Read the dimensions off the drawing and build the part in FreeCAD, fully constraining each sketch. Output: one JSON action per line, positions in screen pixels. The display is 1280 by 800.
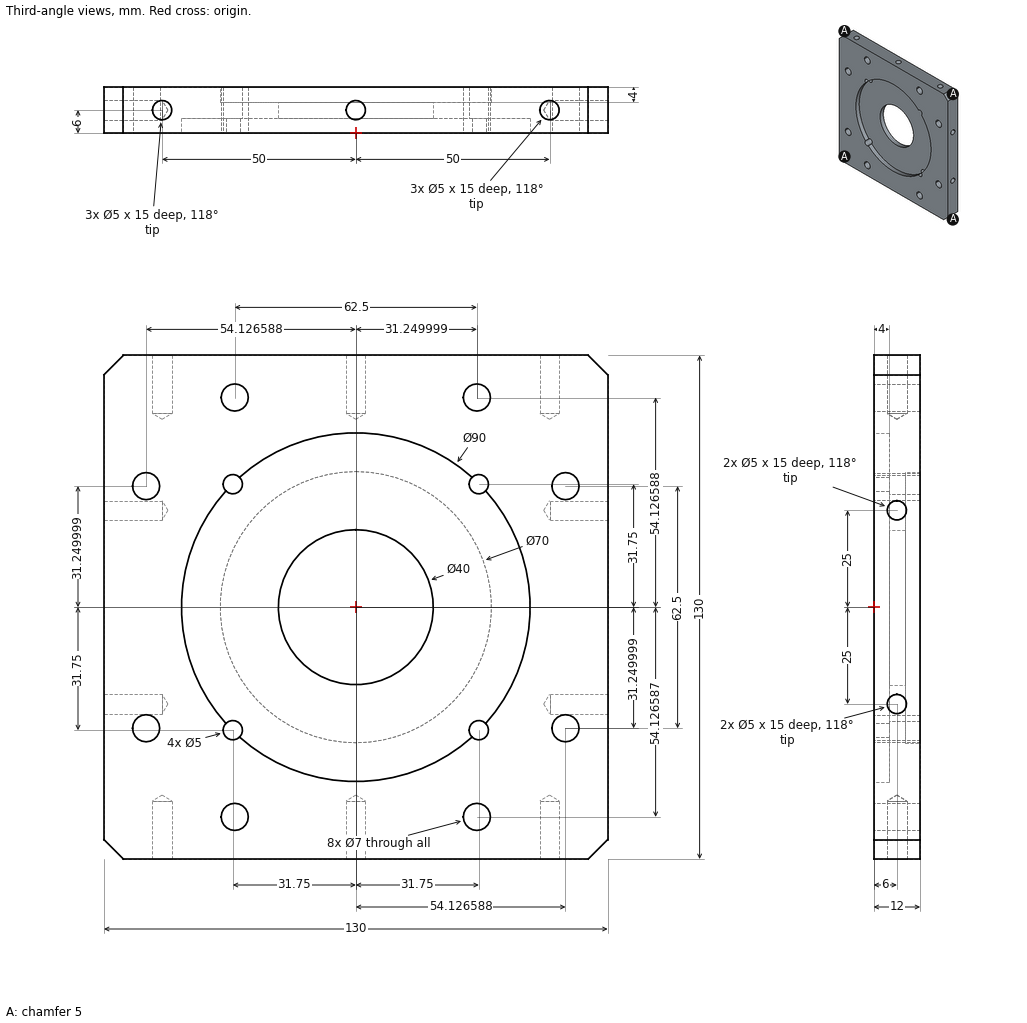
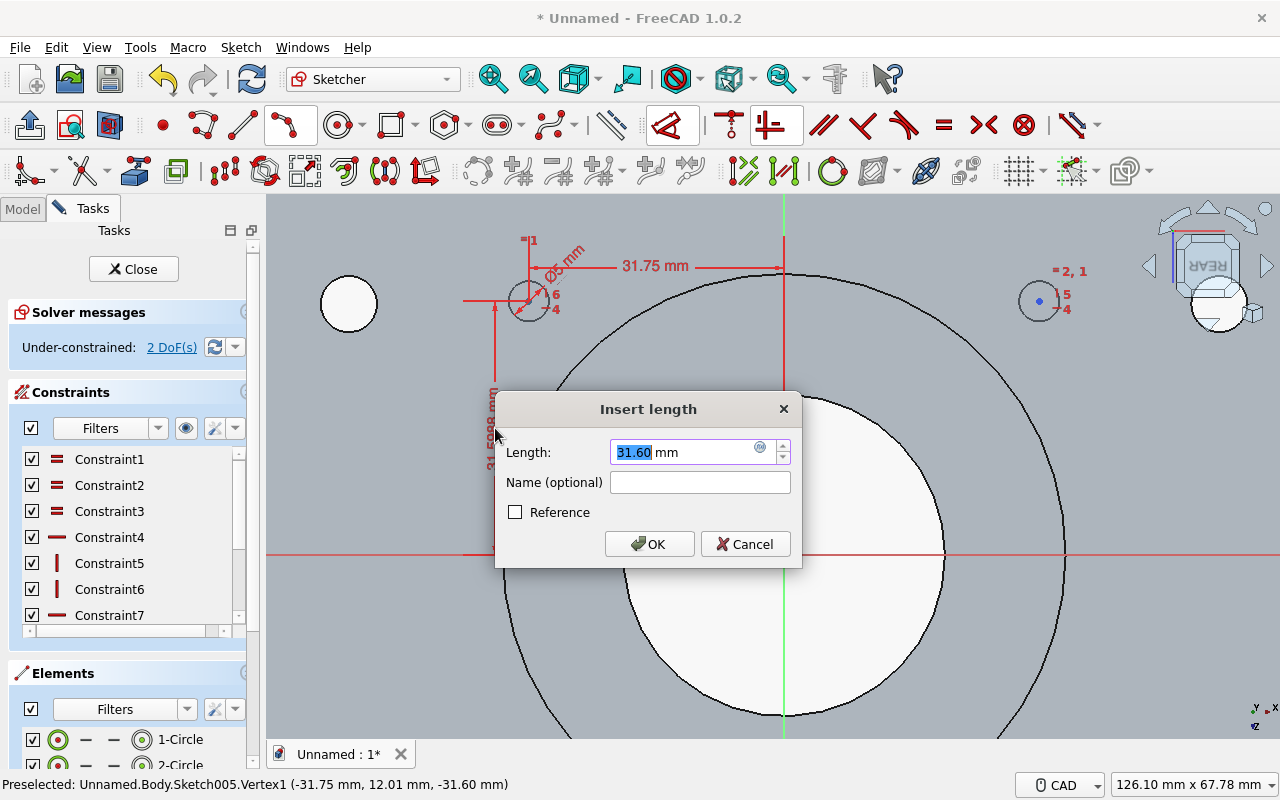
{"action": "type", "text": "31.75"}
{"action": "key", "text": "Return"}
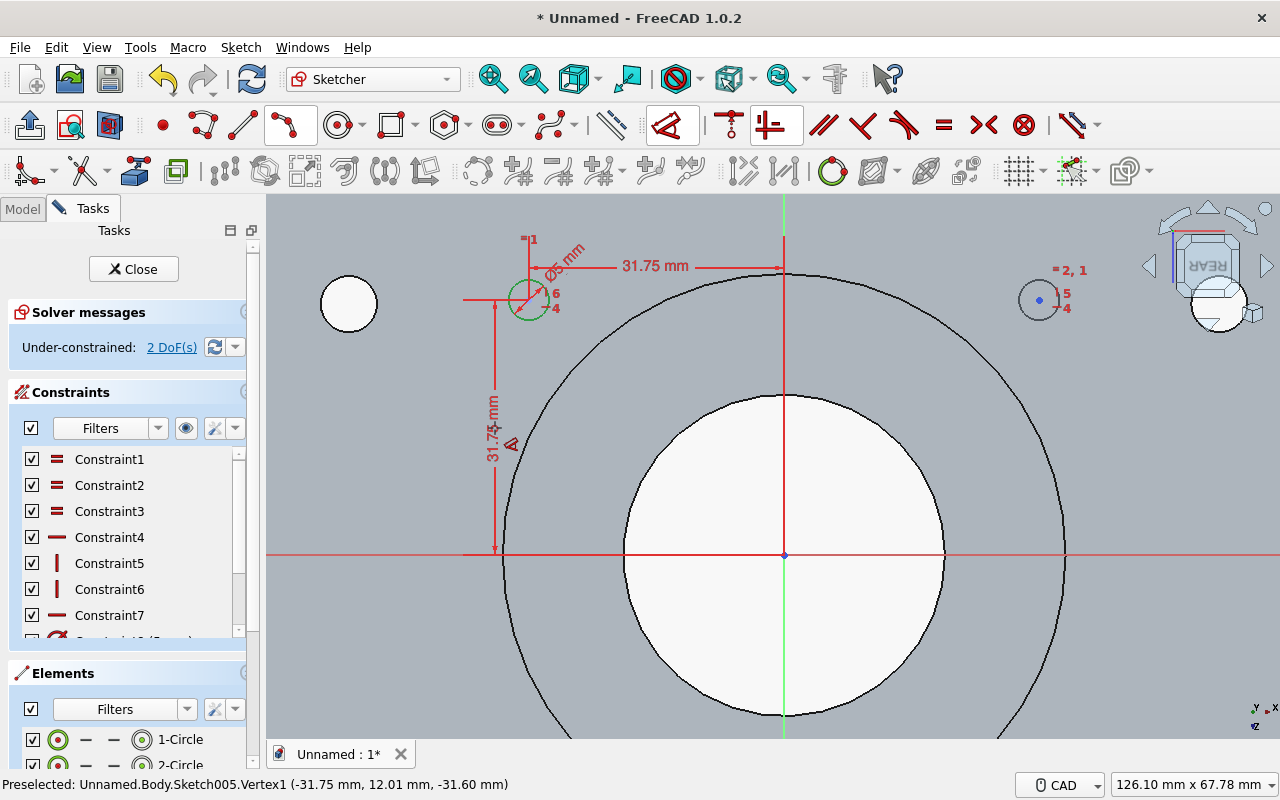
{"action": "left_click", "coordinate": [1039, 300]}
{"action": "left_click", "coordinate": [912, 266]}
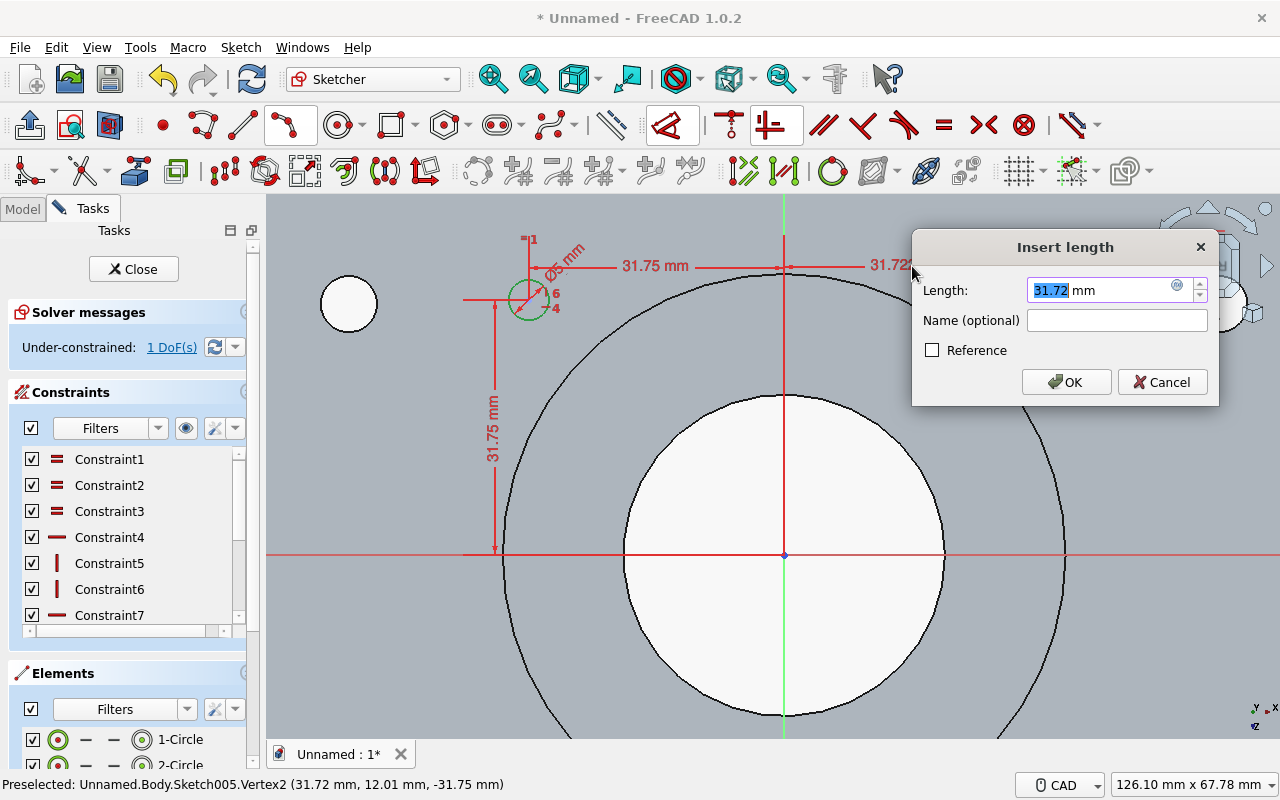
{"action": "type", "text": "31.75"}
{"action": "key", "text": "Return"}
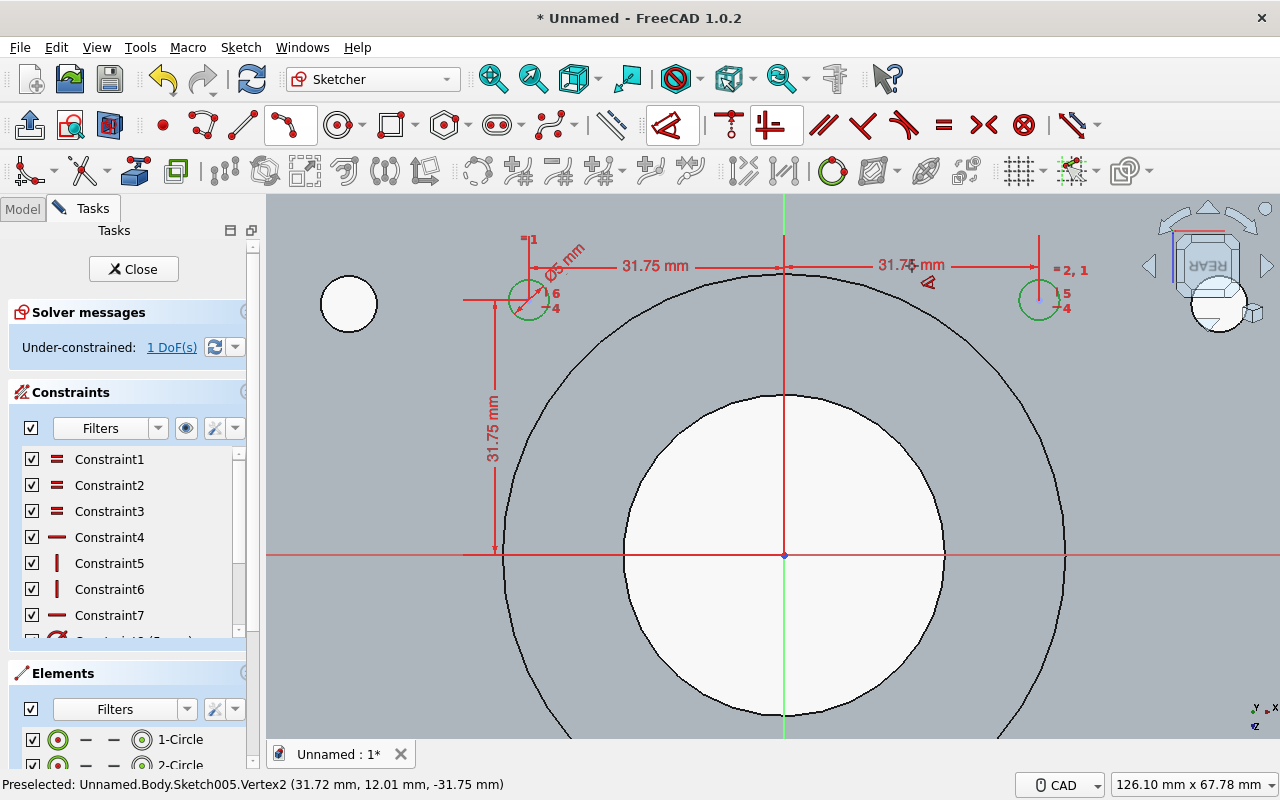
{"action": "scroll", "coordinate": [543, 286], "scroll_direction": "down", "scroll_amount": 2}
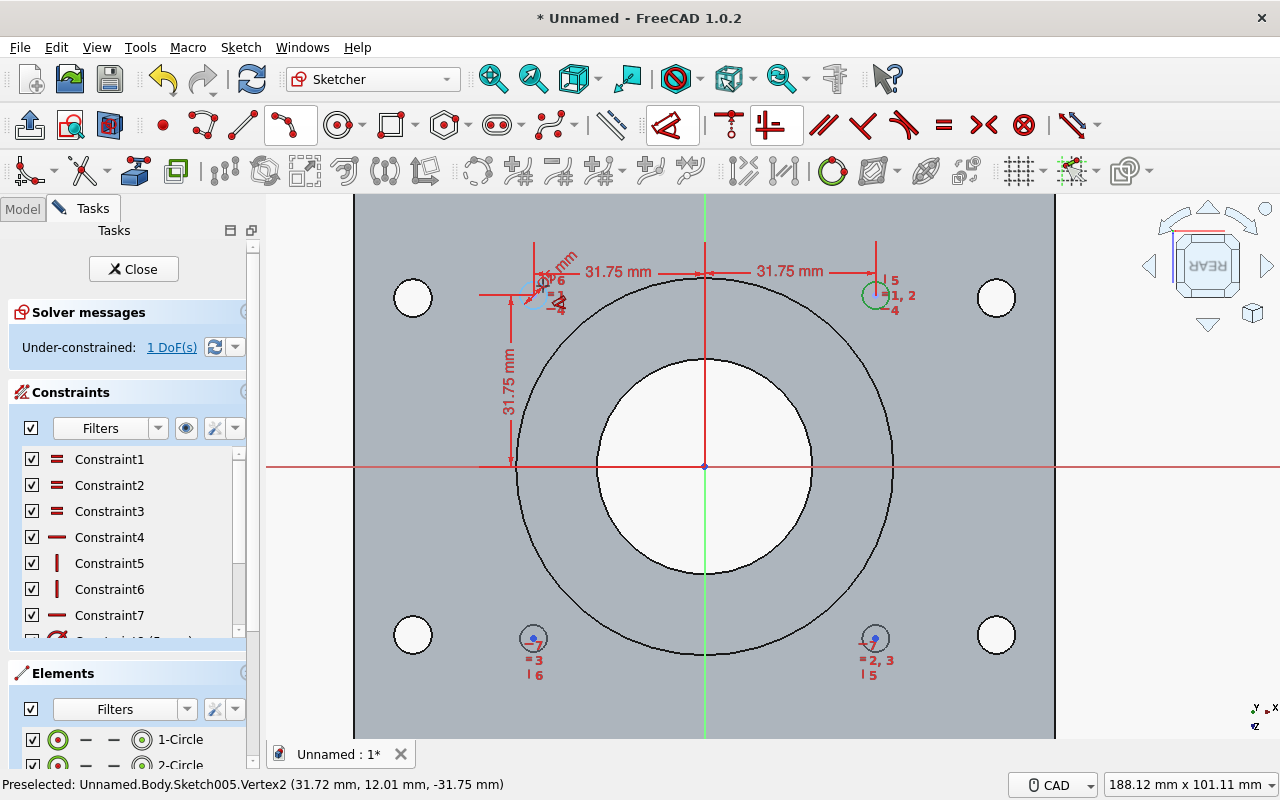
{"action": "left_click", "coordinate": [876, 638]}
{"action": "left_click", "coordinate": [910, 553]}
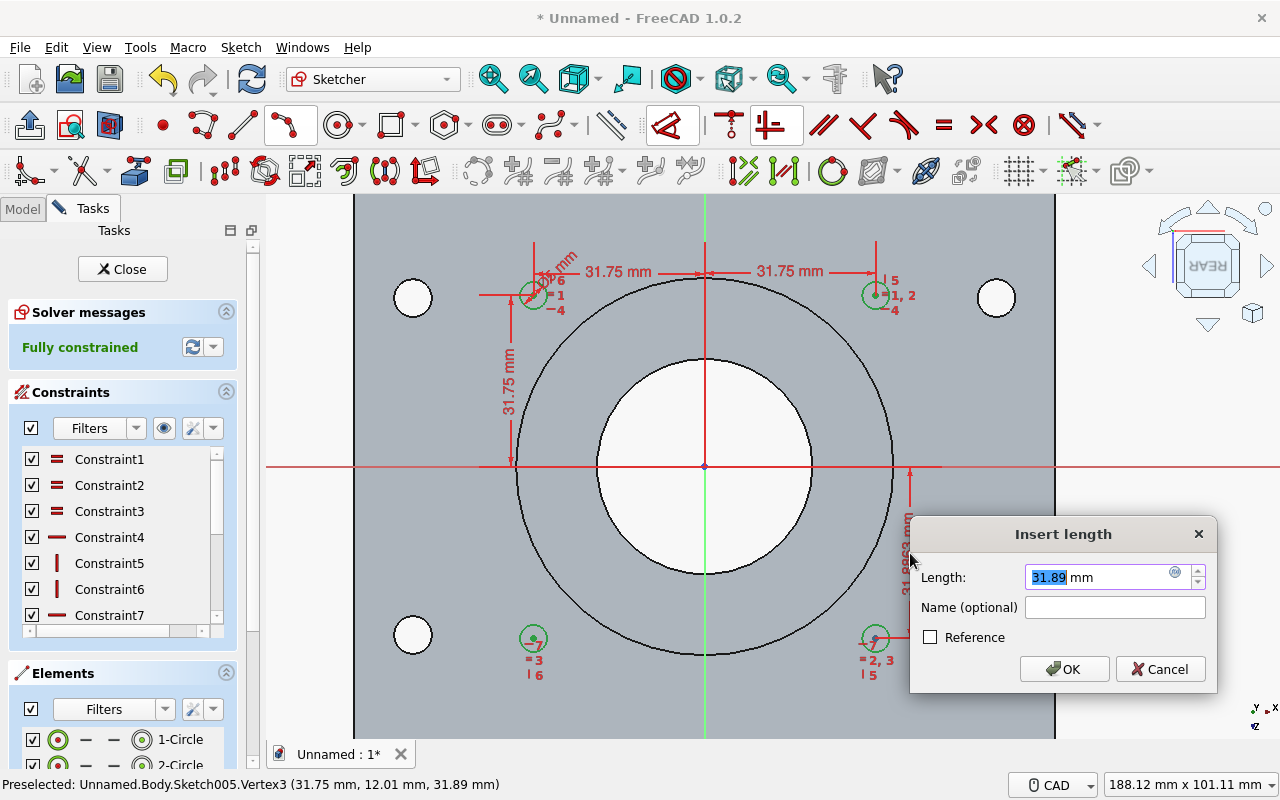
{"action": "type", "text": "31.75"}
{"action": "key", "text": "Return"}
{"action": "key", "text": "Escape"}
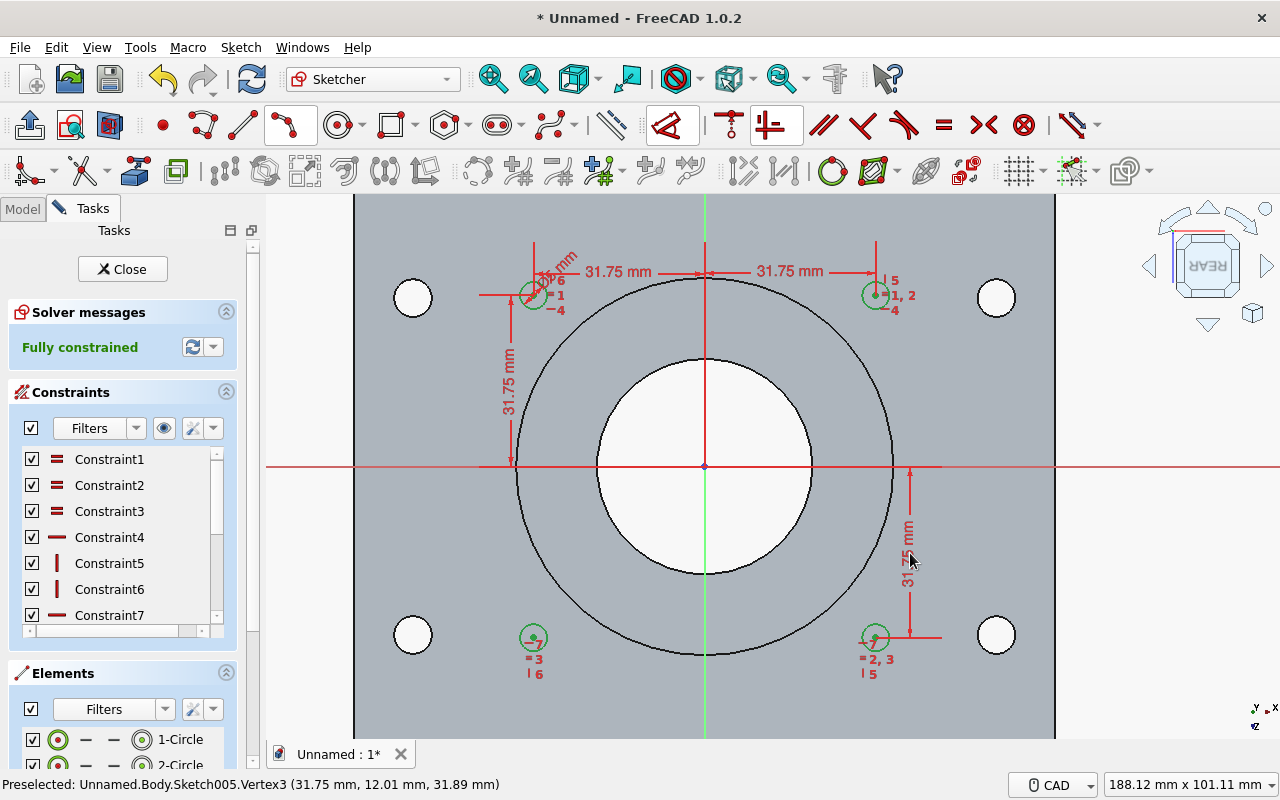
{"action": "left_click", "coordinate": [123, 269]}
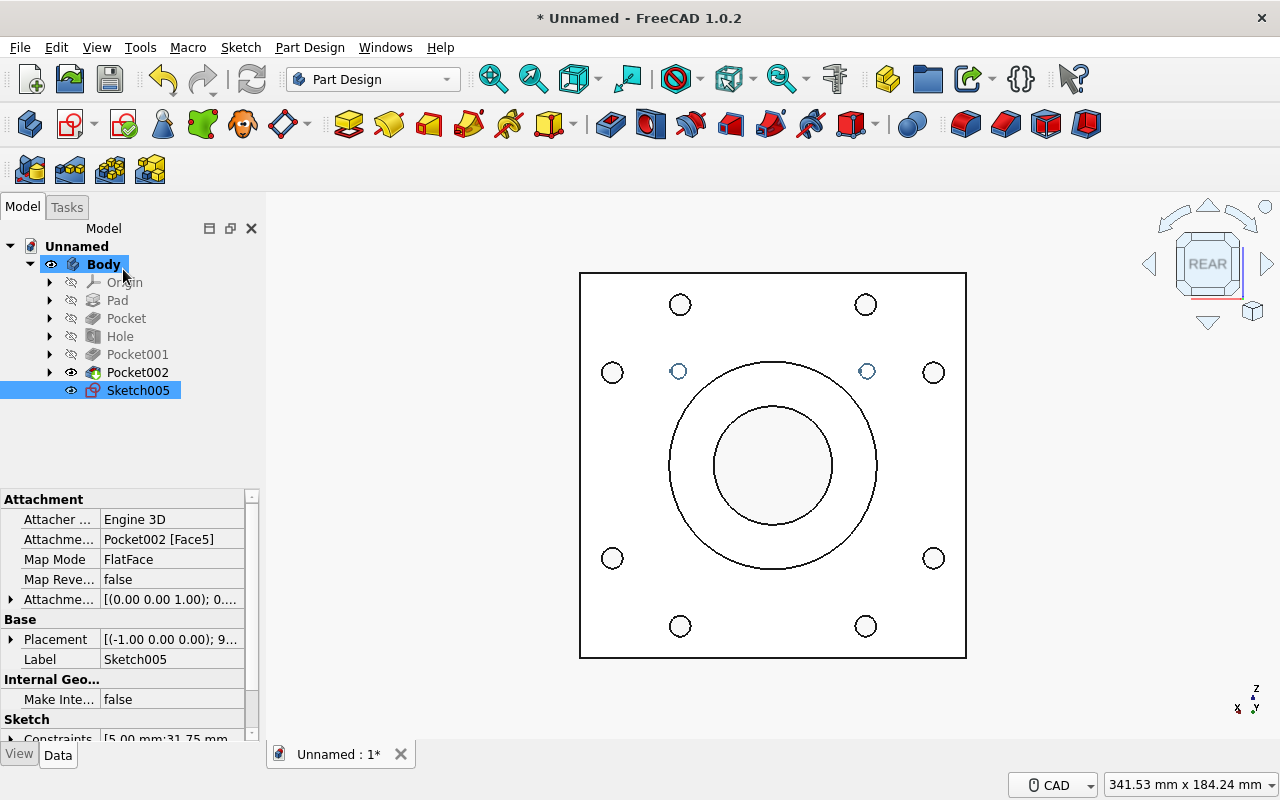
{"action": "left_click", "coordinate": [612, 124]}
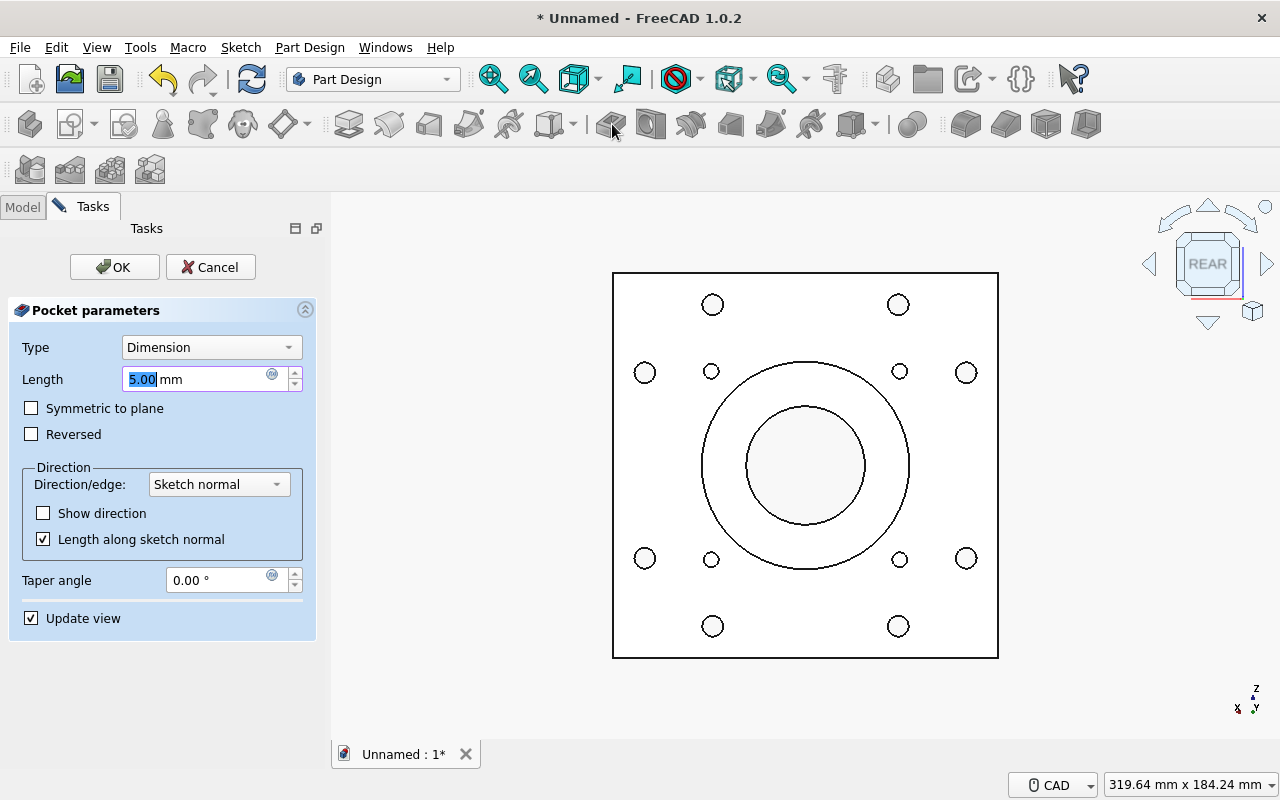
{"action": "left_click", "coordinate": [212, 348]}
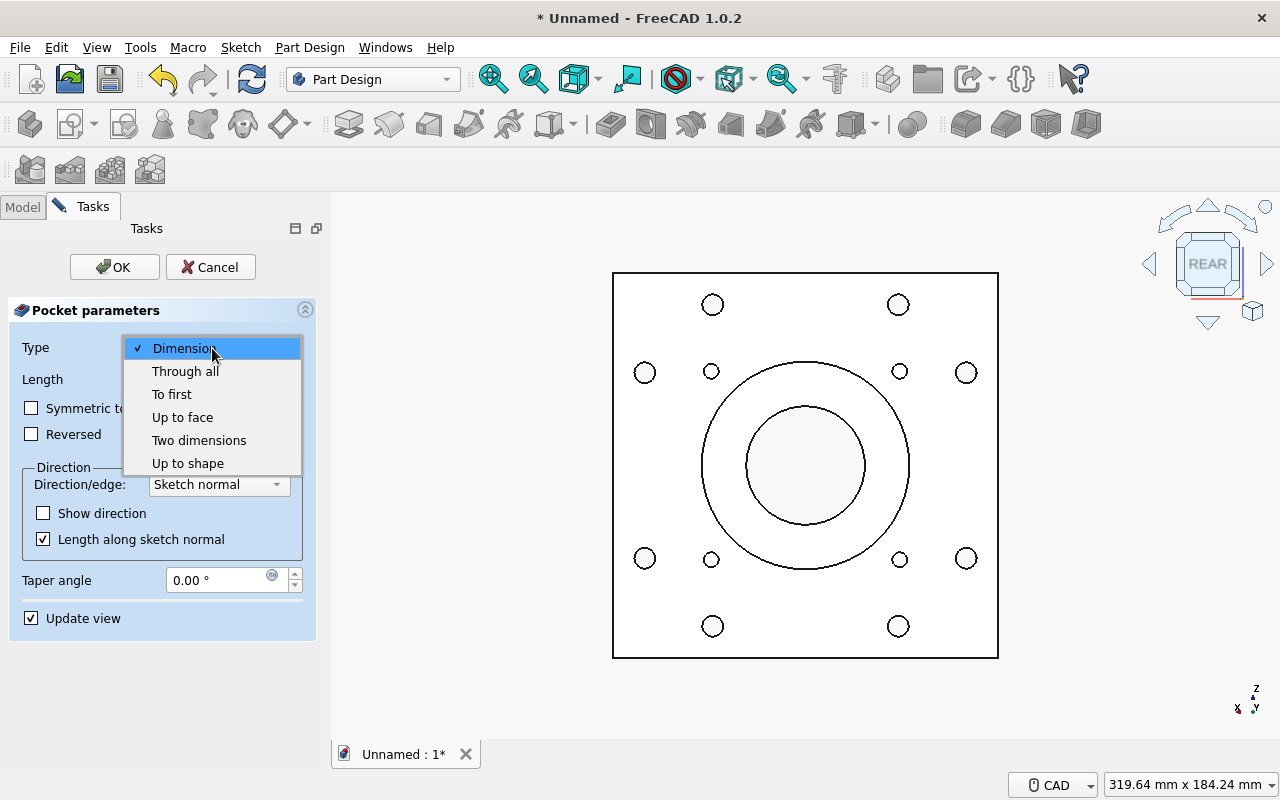
{"action": "left_click", "coordinate": [212, 372]}